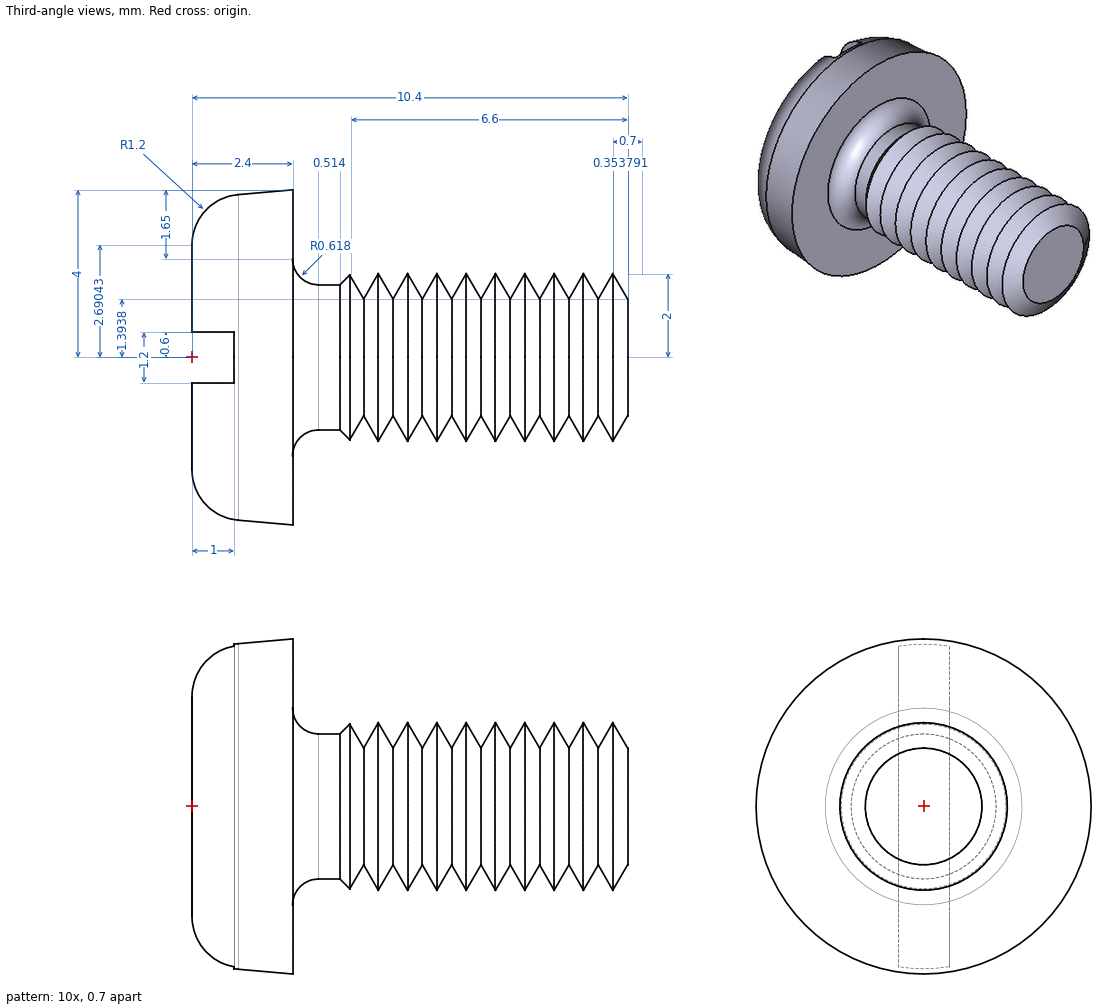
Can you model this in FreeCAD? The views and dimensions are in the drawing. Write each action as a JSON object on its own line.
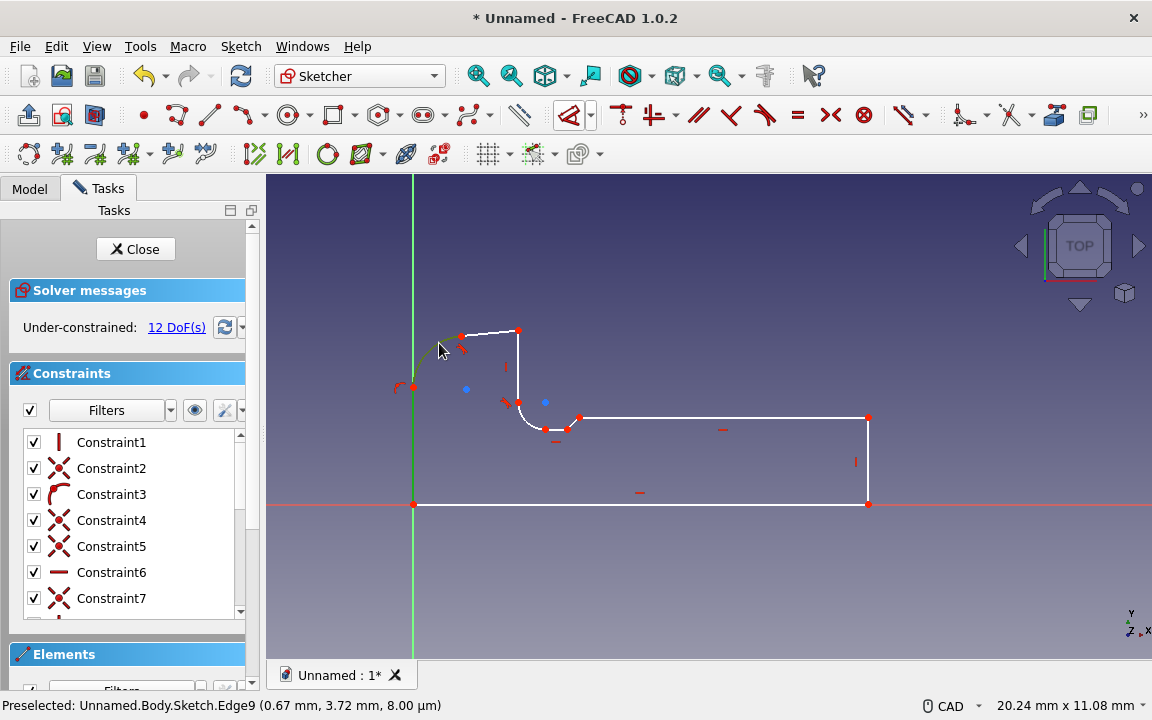
{"action": "left_click", "coordinate": [765, 116]}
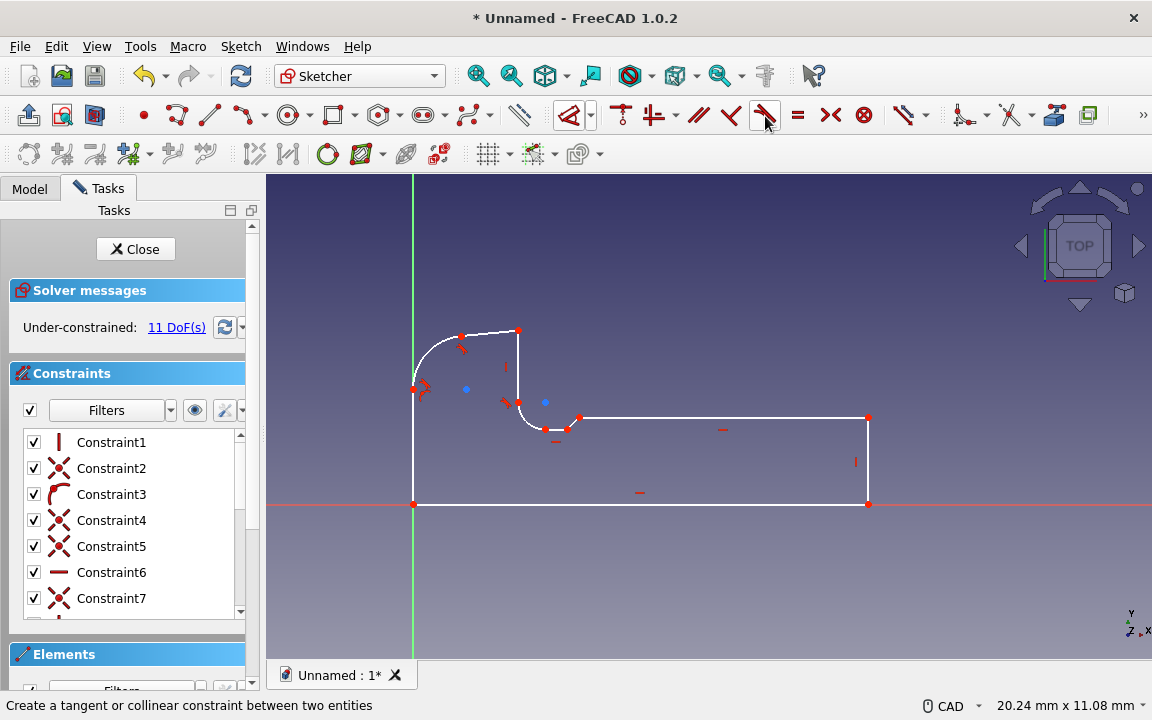
{"action": "scroll", "coordinate": [556, 430], "scroll_direction": "up", "scroll_amount": 2}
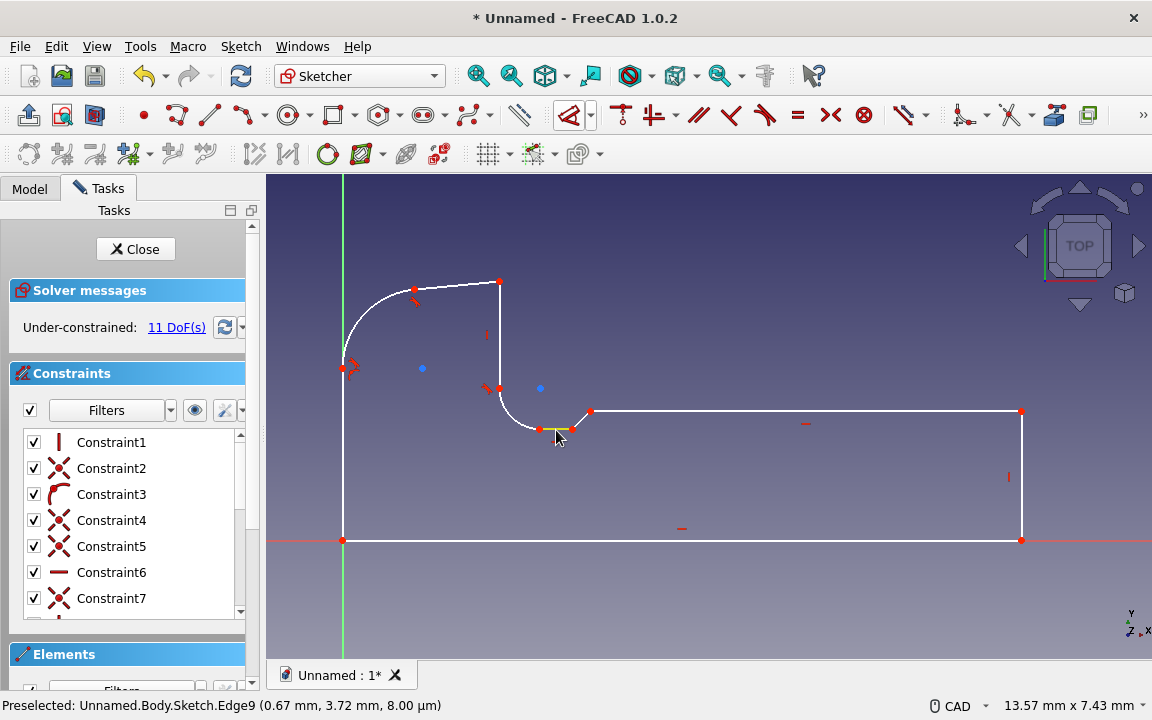
{"action": "left_click", "coordinate": [556, 429]}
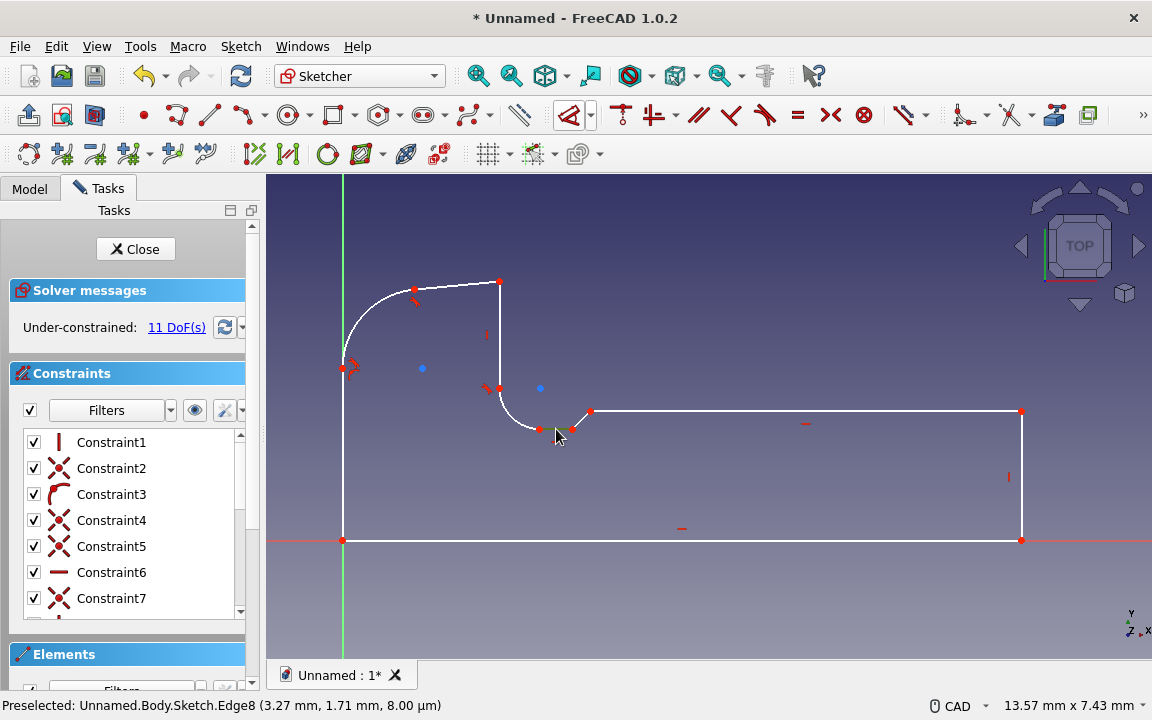
{"action": "left_click", "coordinate": [504, 407]}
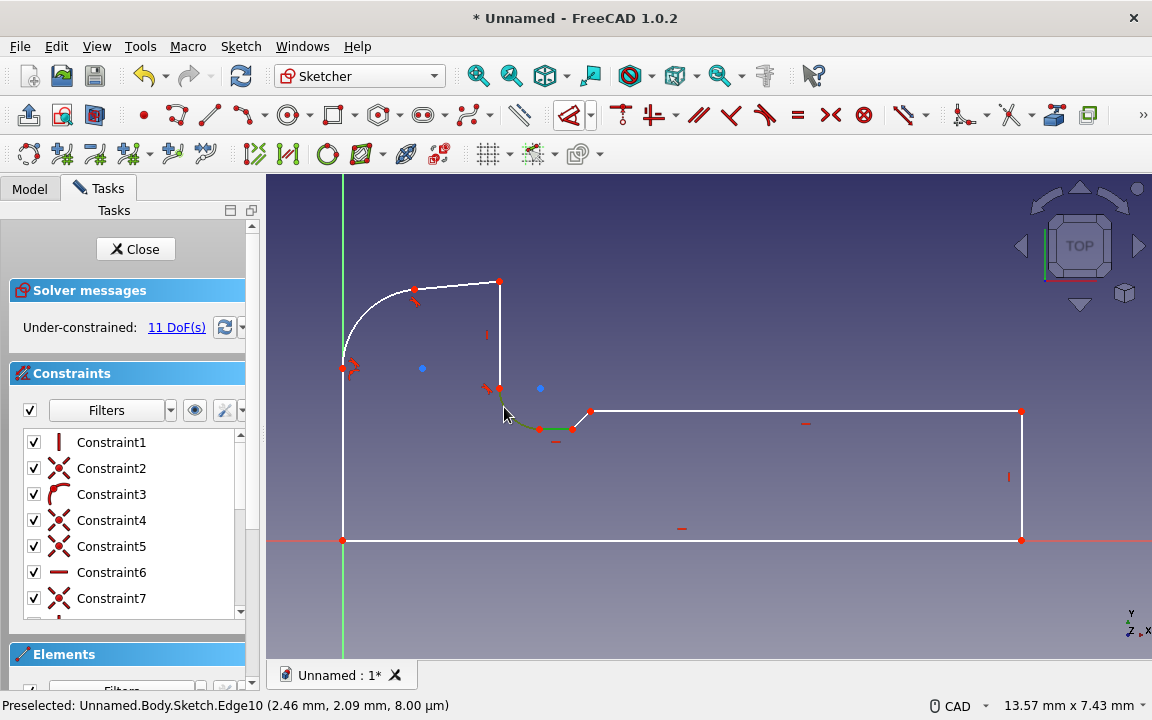
{"action": "left_click", "coordinate": [765, 116]}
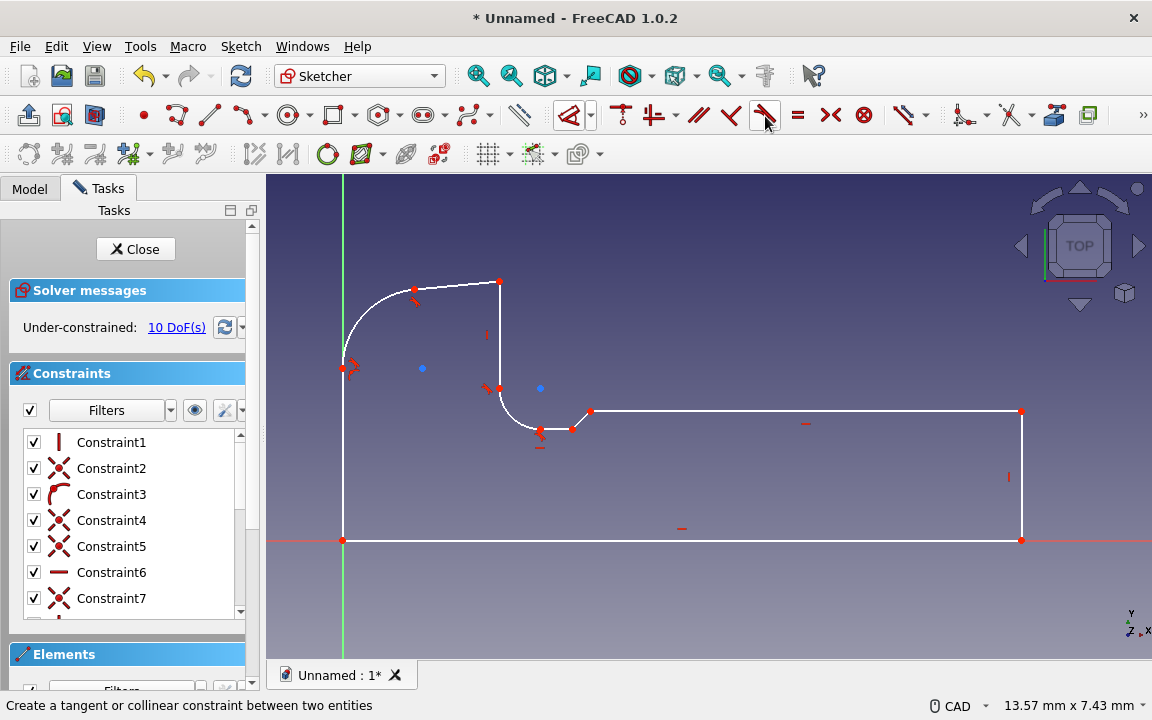
{"action": "left_click", "coordinate": [568, 116]}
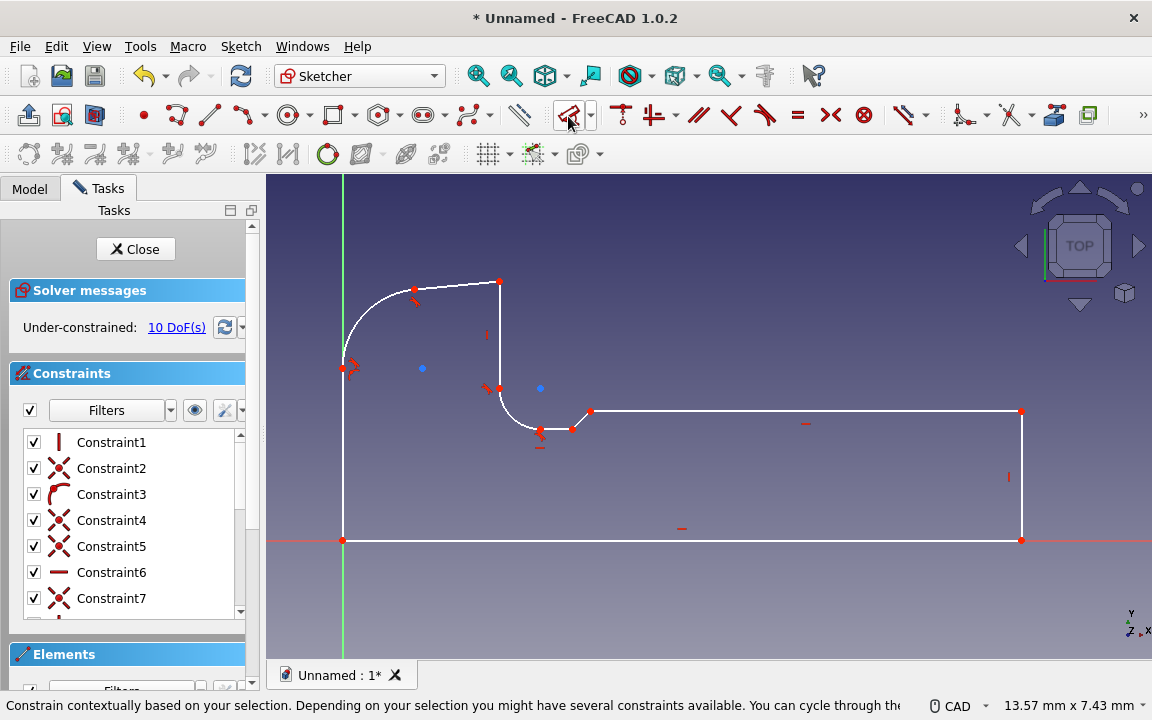
{"action": "left_click", "coordinate": [381, 300]}
{"action": "left_click", "coordinate": [365, 273]}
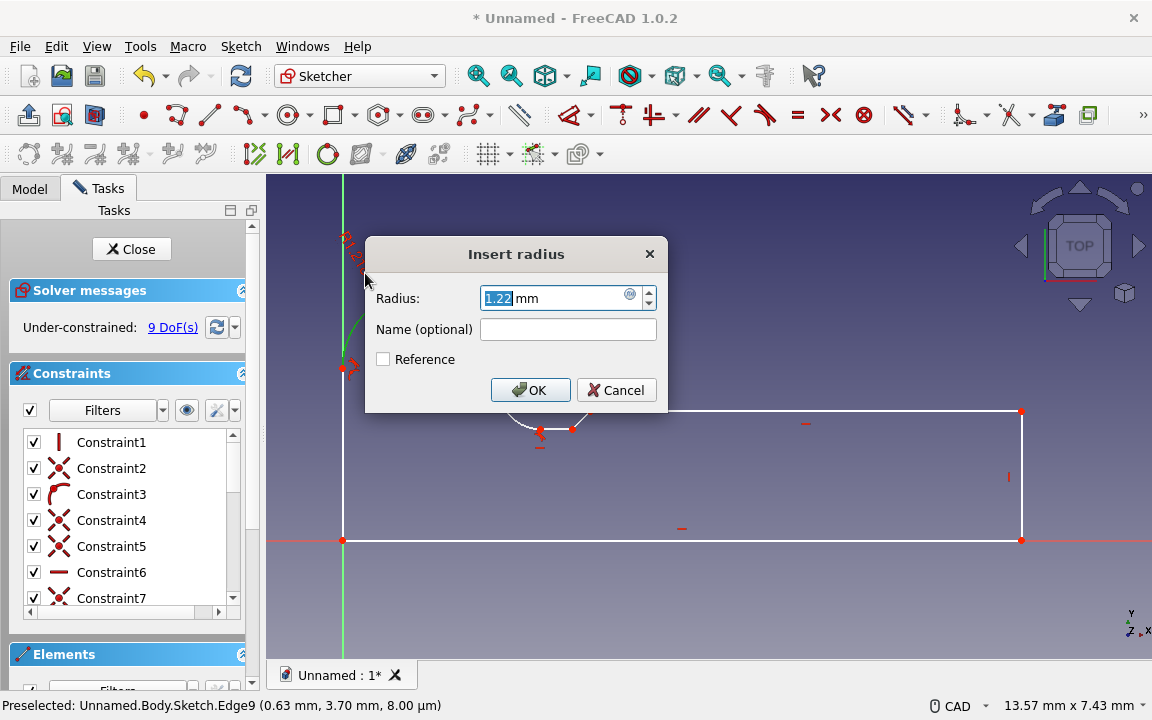
{"action": "type", "text": "1.2"}
{"action": "key", "text": "Return"}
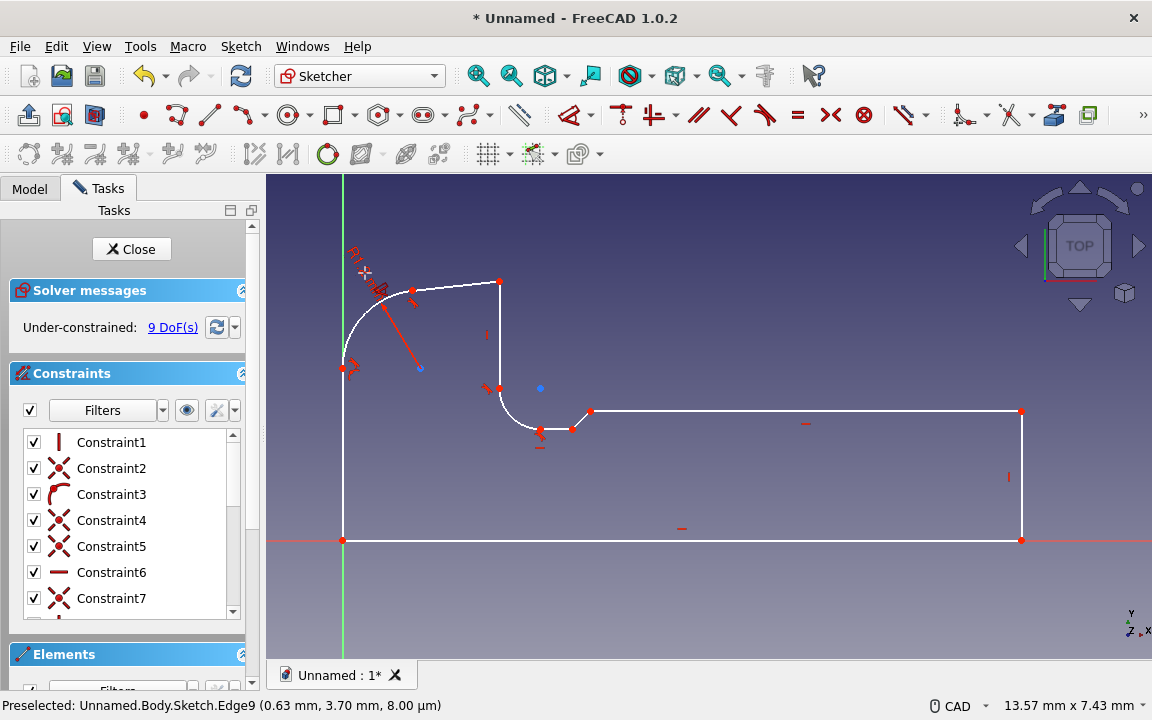
{"action": "left_click", "coordinate": [504, 407]}
{"action": "left_click", "coordinate": [476, 422]}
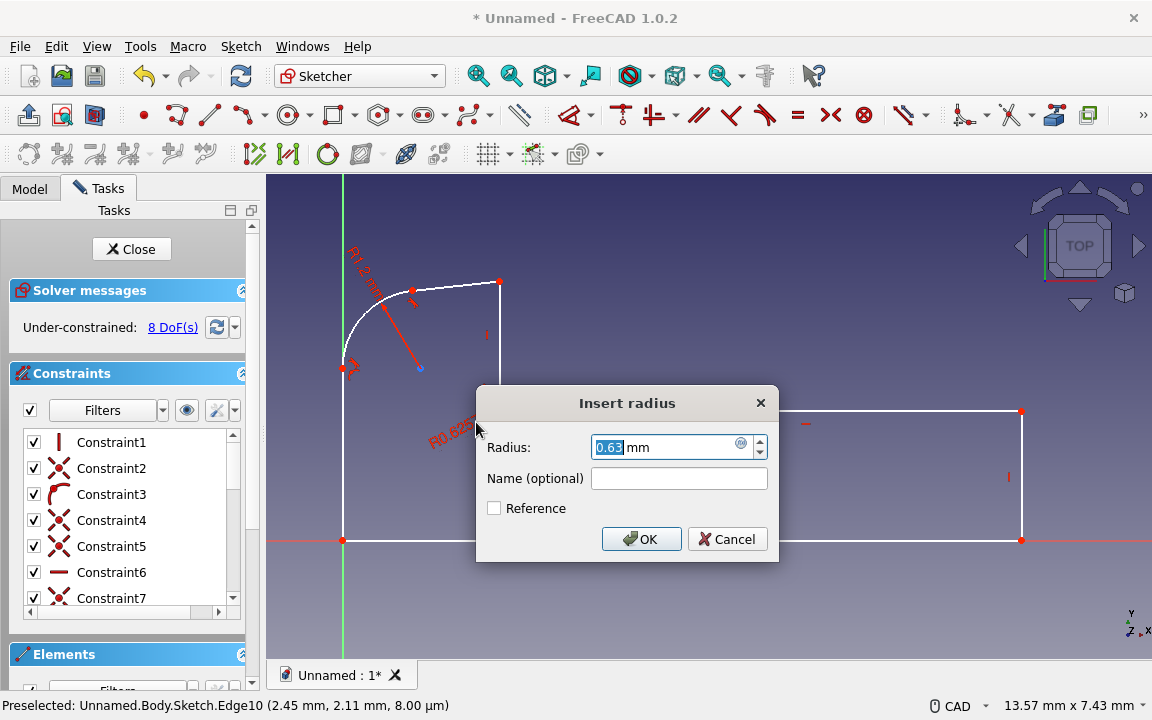
{"action": "type", "text": "0.618"}
{"action": "key", "text": "Return"}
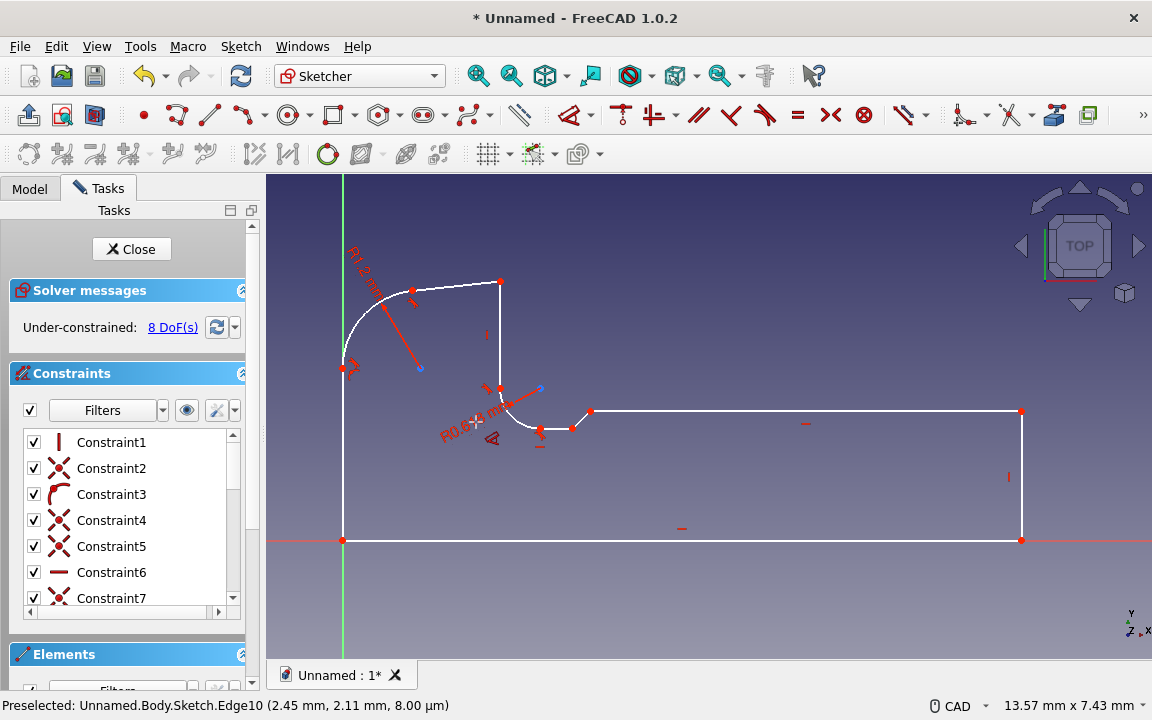
{"action": "scroll", "coordinate": [556, 429], "scroll_direction": "down", "scroll_amount": 2}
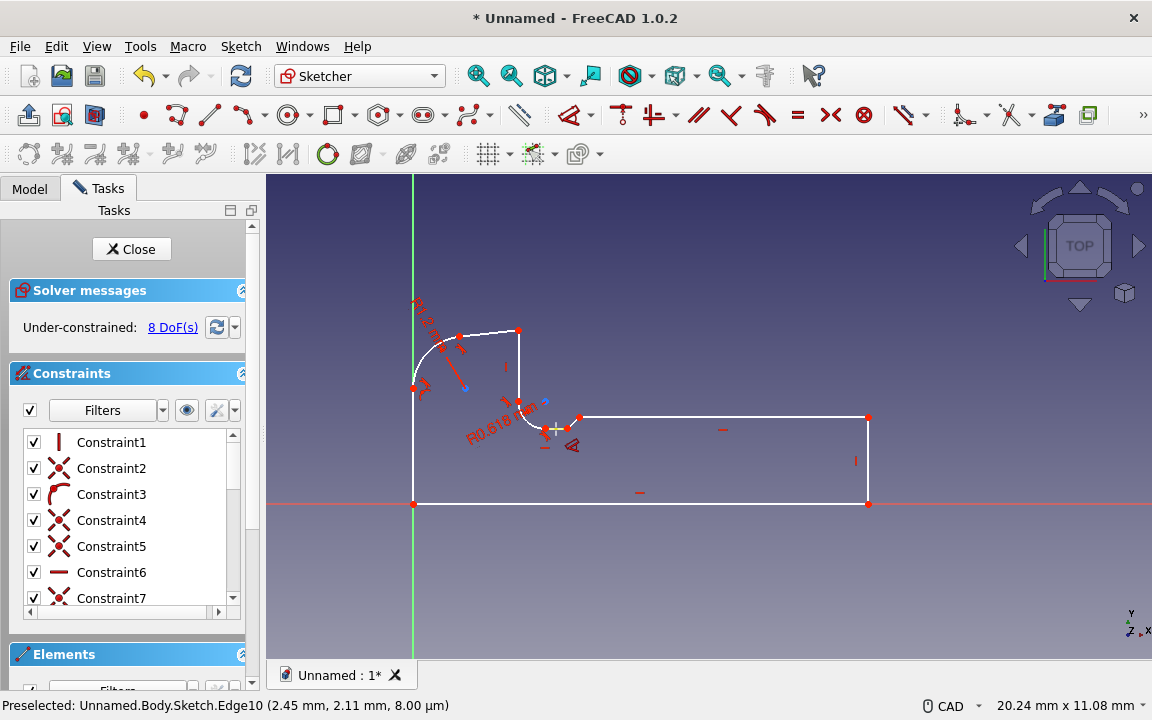
{"action": "left_click", "coordinate": [868, 478]}
{"action": "left_click", "coordinate": [902, 461]}